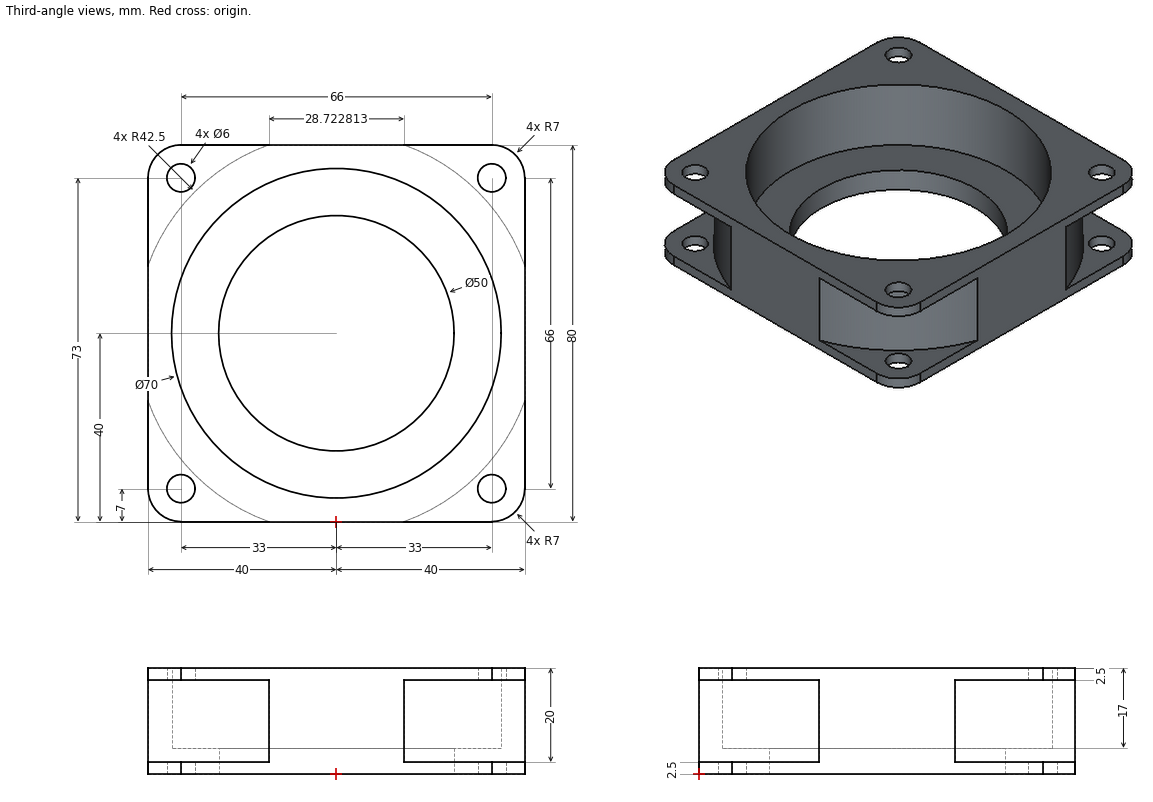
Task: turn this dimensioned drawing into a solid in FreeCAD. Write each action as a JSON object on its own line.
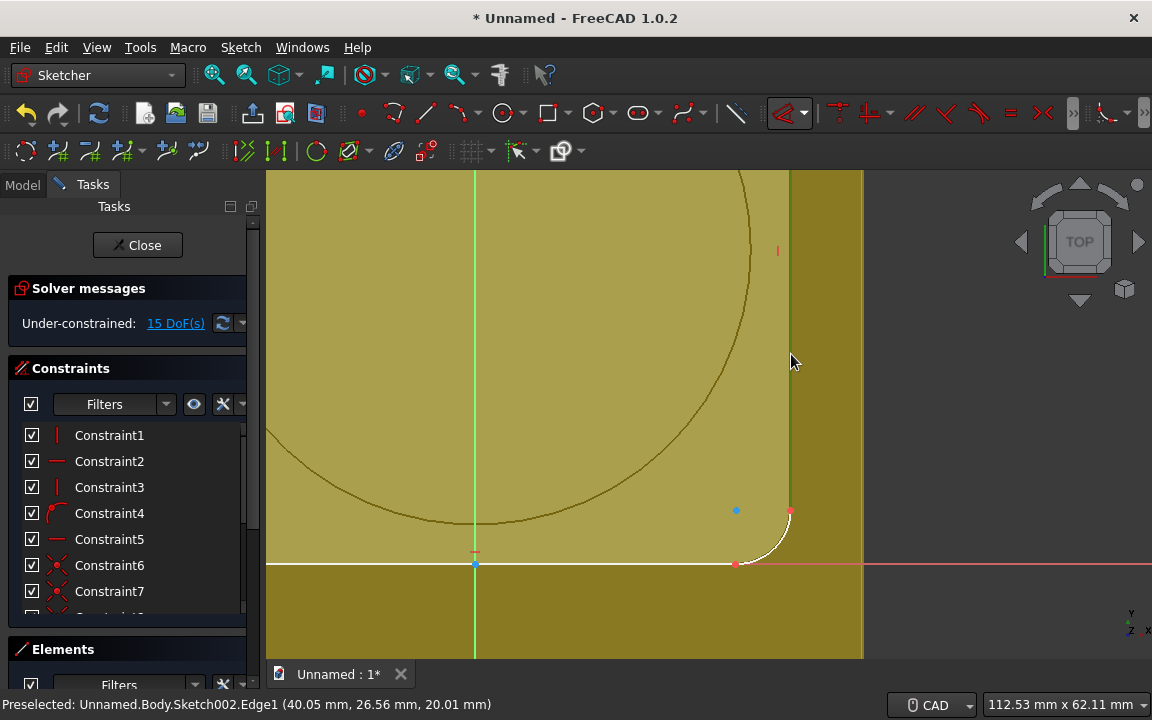
{"action": "scroll", "coordinate": [775, 549], "scroll_direction": "down", "scroll_amount": 4}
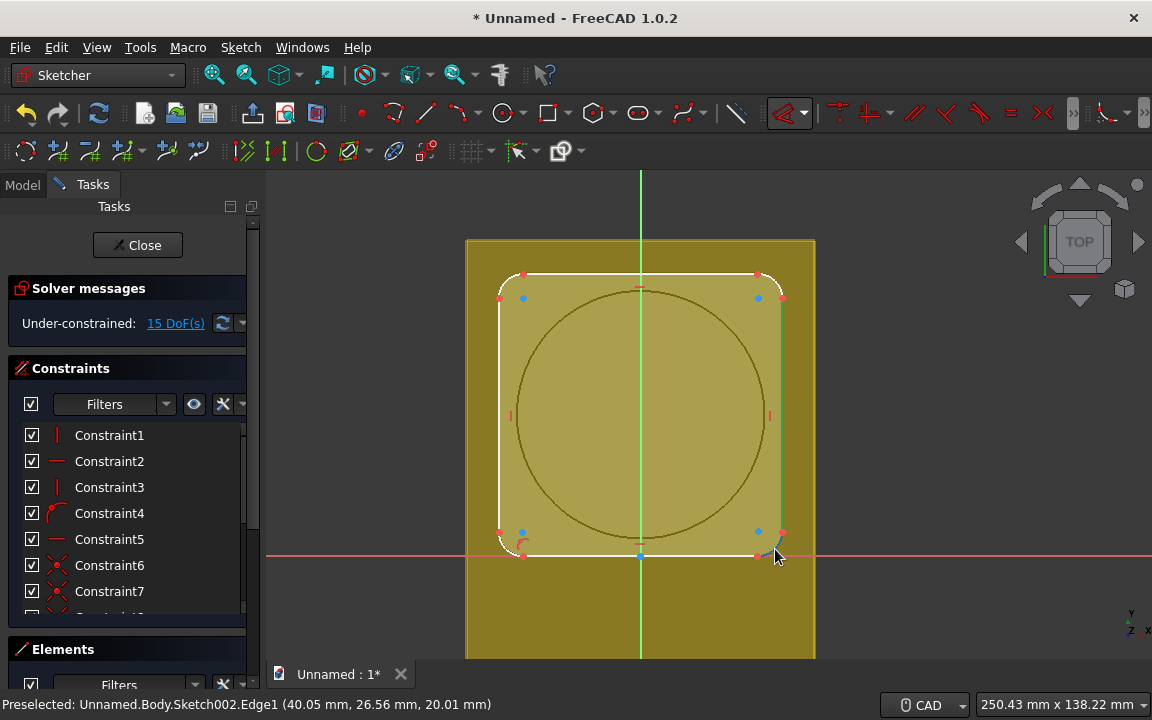
{"action": "left_click", "coordinate": [780, 287]}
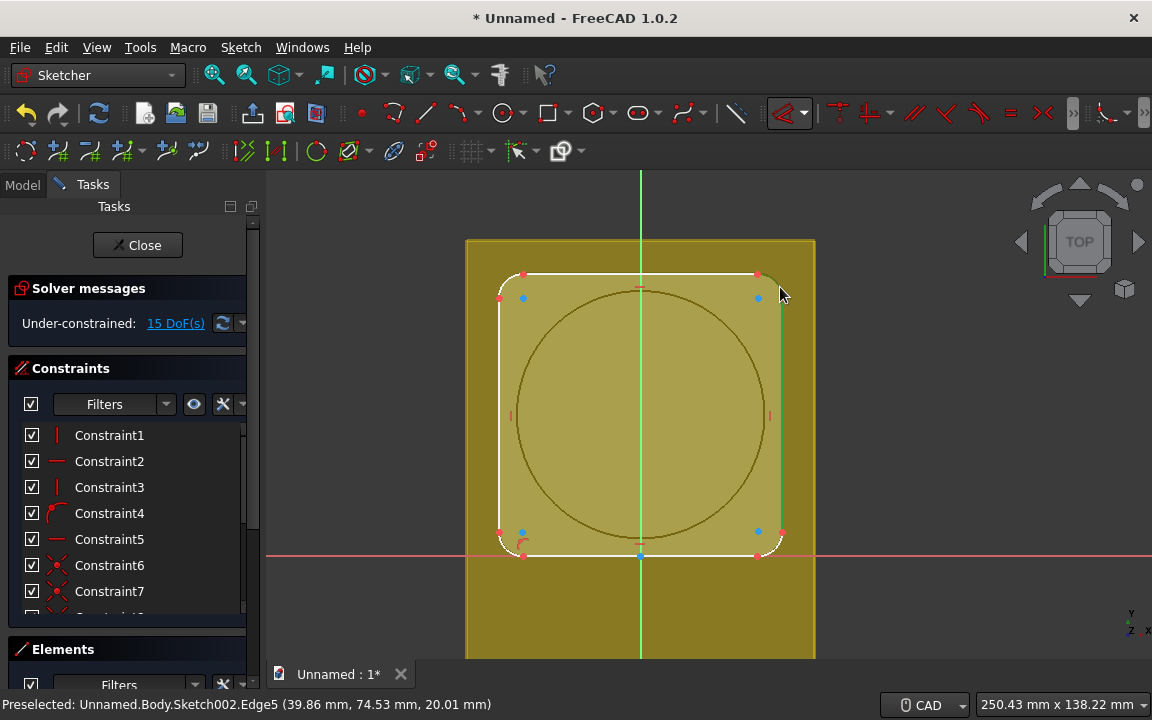
{"action": "left_click", "coordinate": [980, 114]}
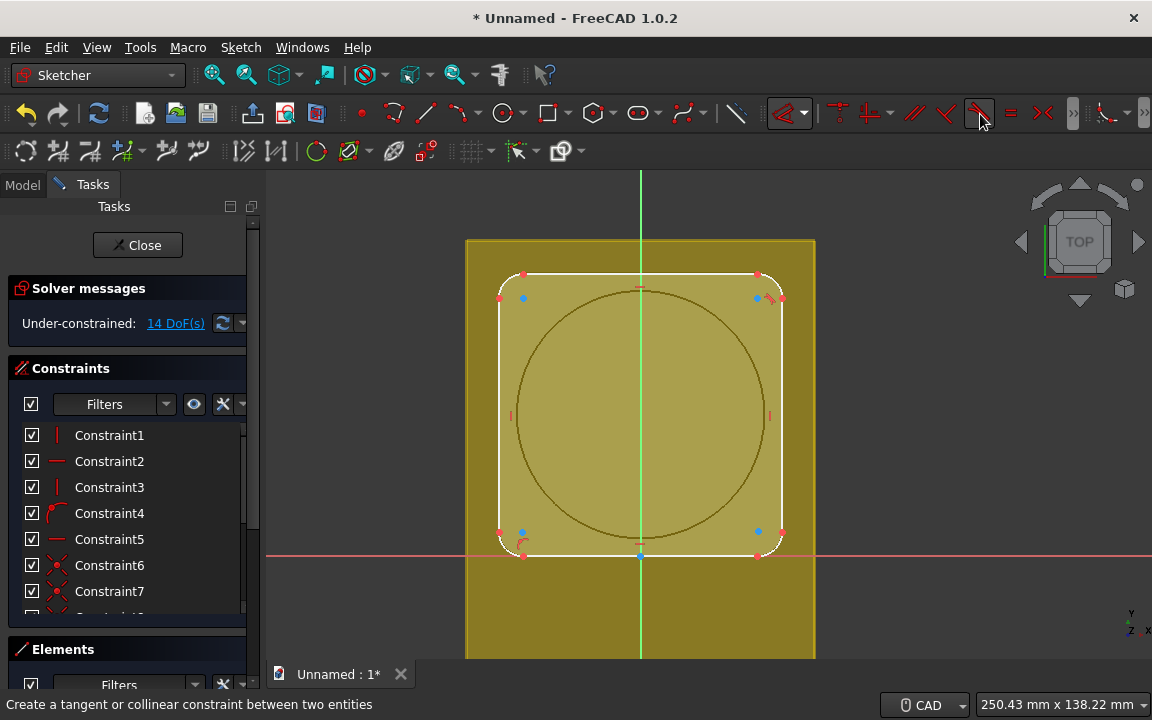
{"action": "left_click", "coordinate": [782, 462]}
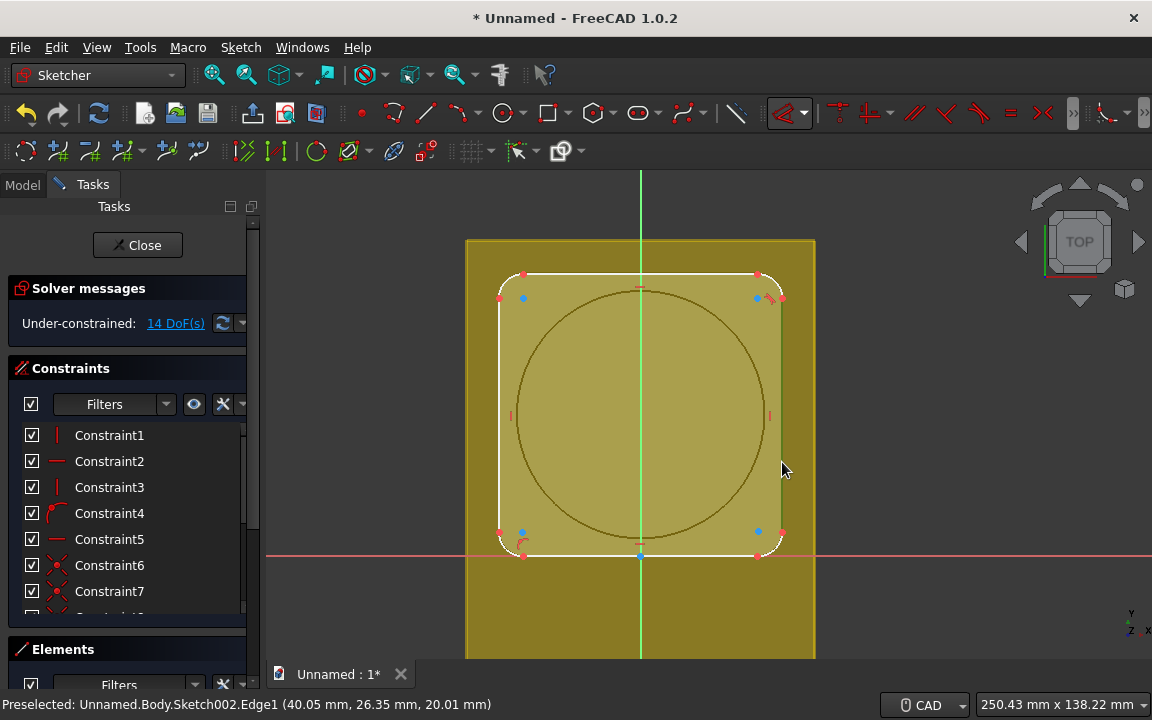
{"action": "left_click", "coordinate": [769, 554]}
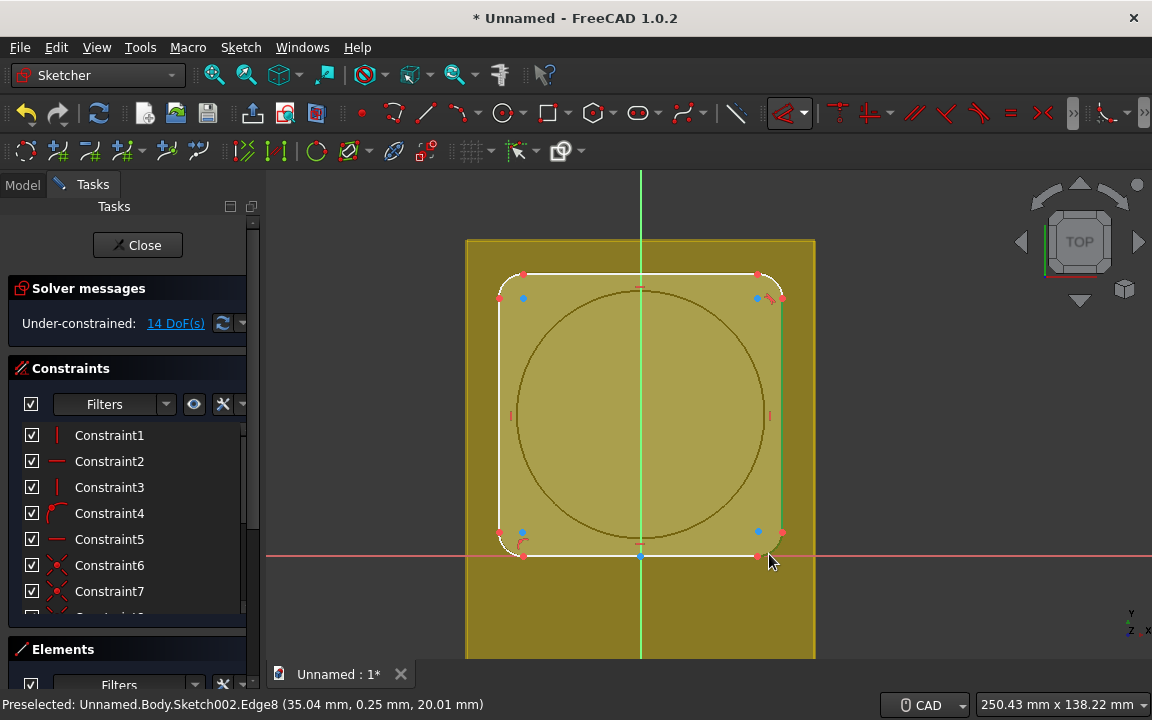
{"action": "left_click", "coordinate": [980, 114]}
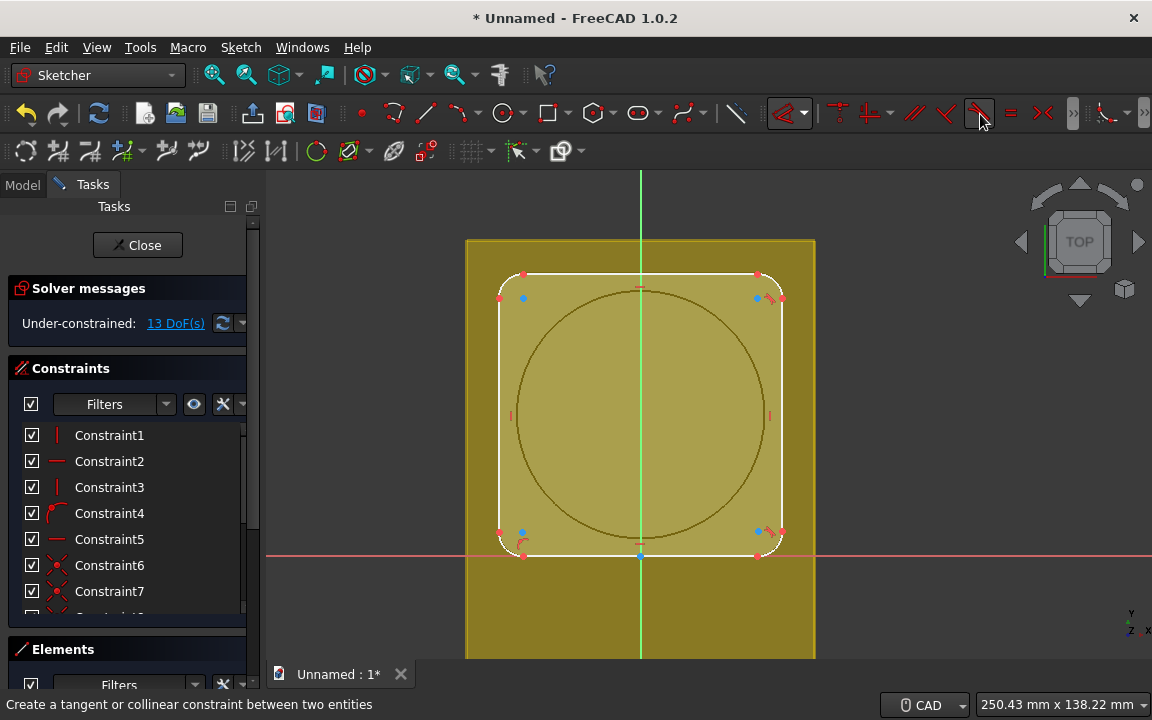
{"action": "left_click", "coordinate": [688, 274]}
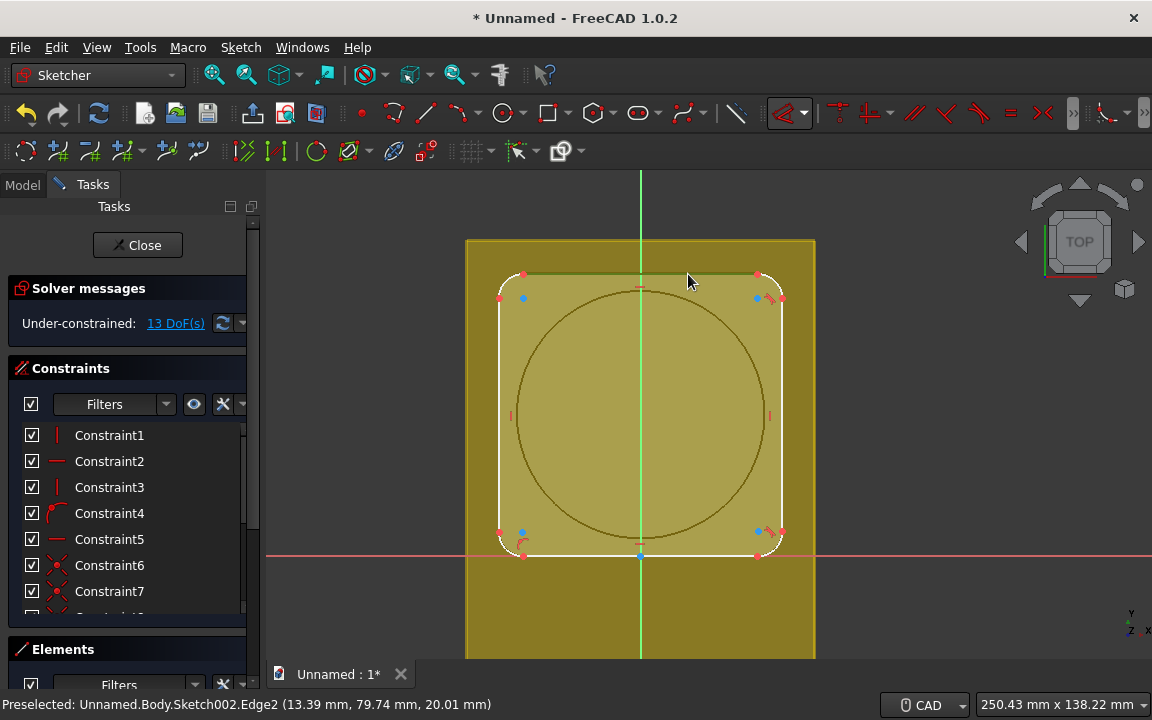
{"action": "left_click", "coordinate": [780, 288]}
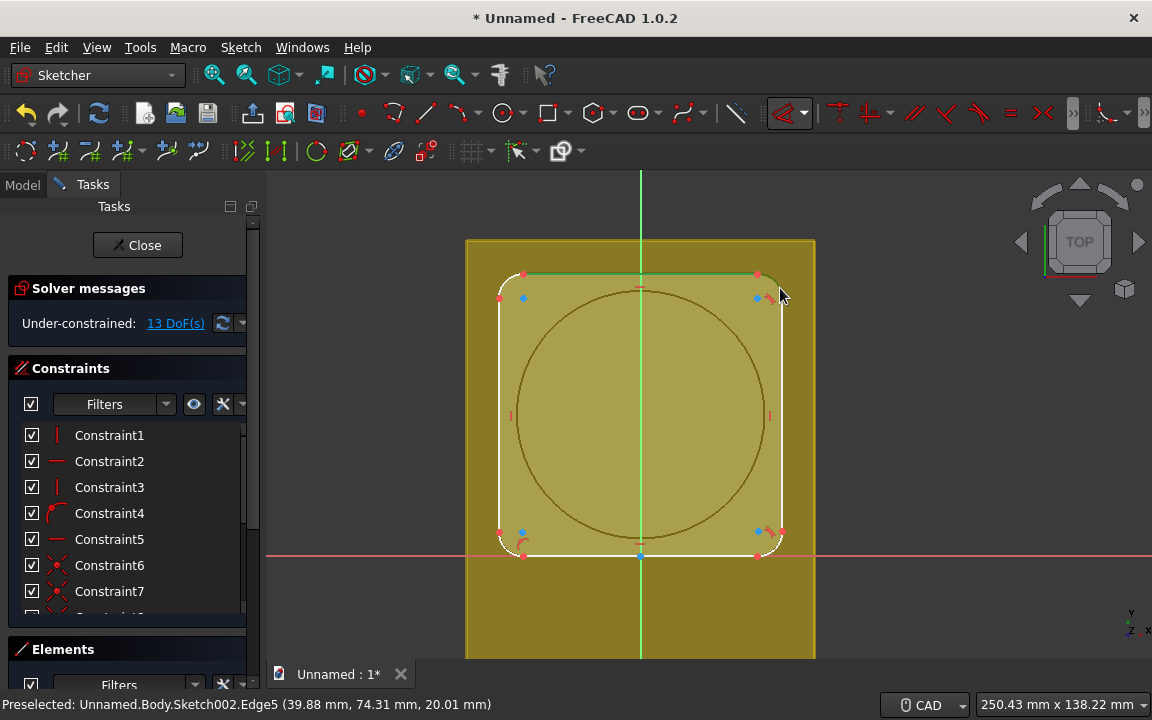
{"action": "key", "text": "t"}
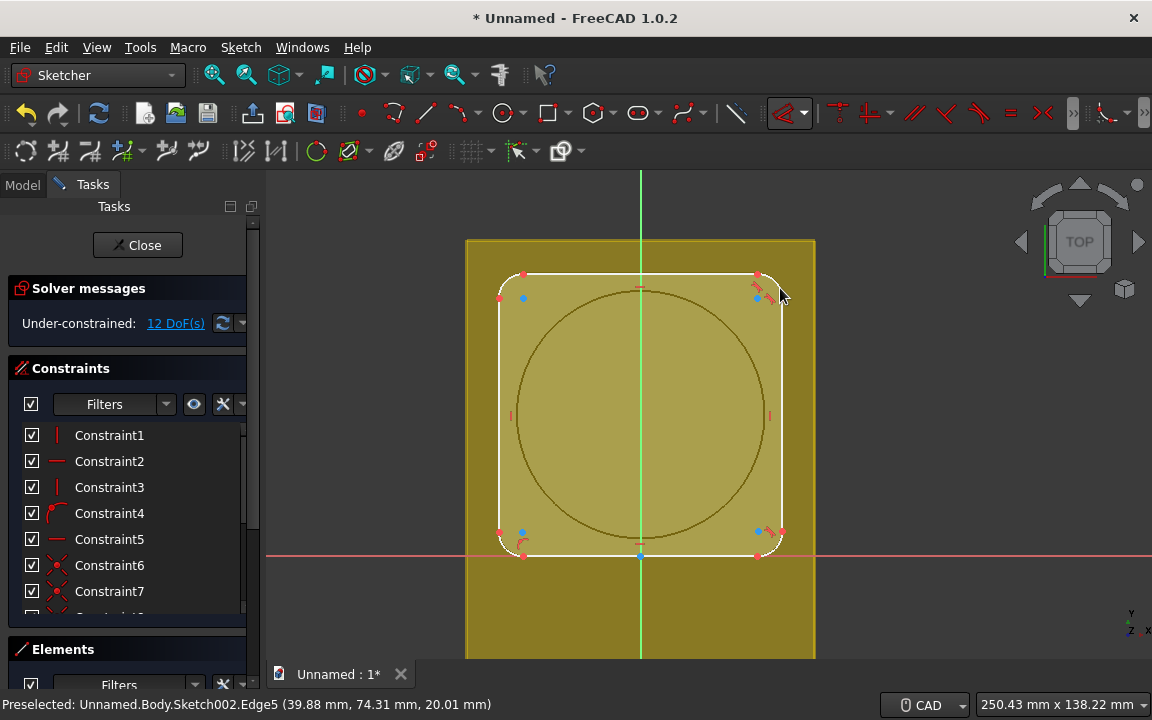
{"action": "left_click", "coordinate": [688, 274]}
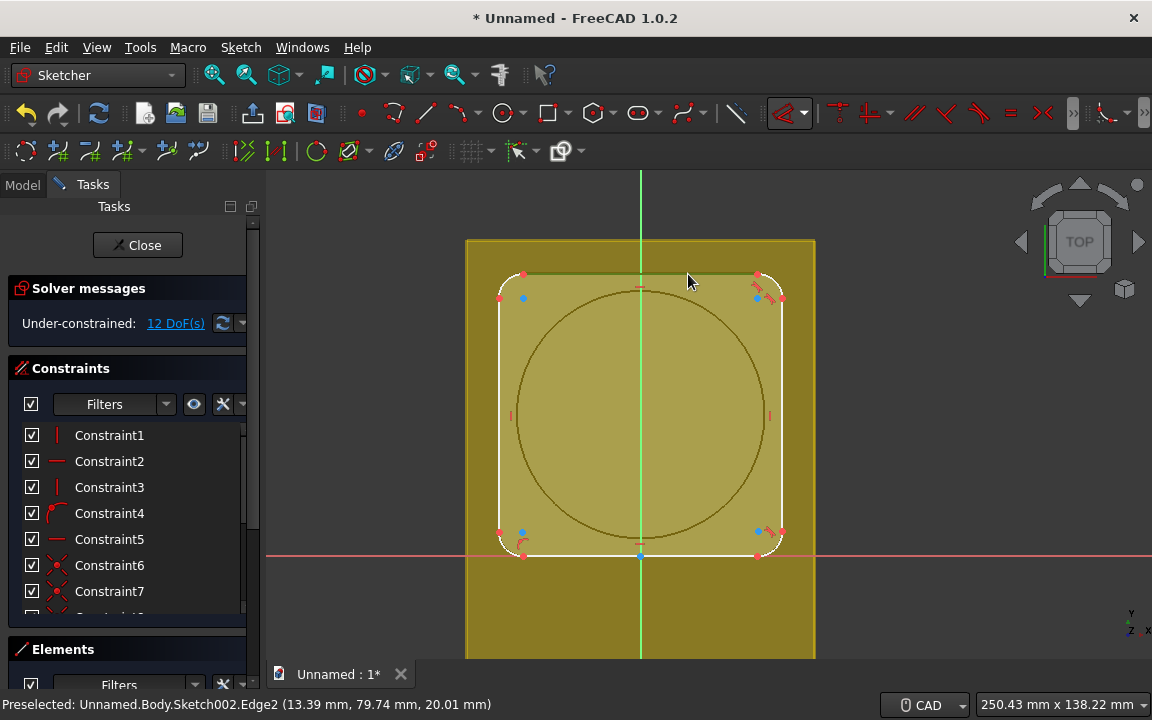
{"action": "left_click", "coordinate": [512, 277]}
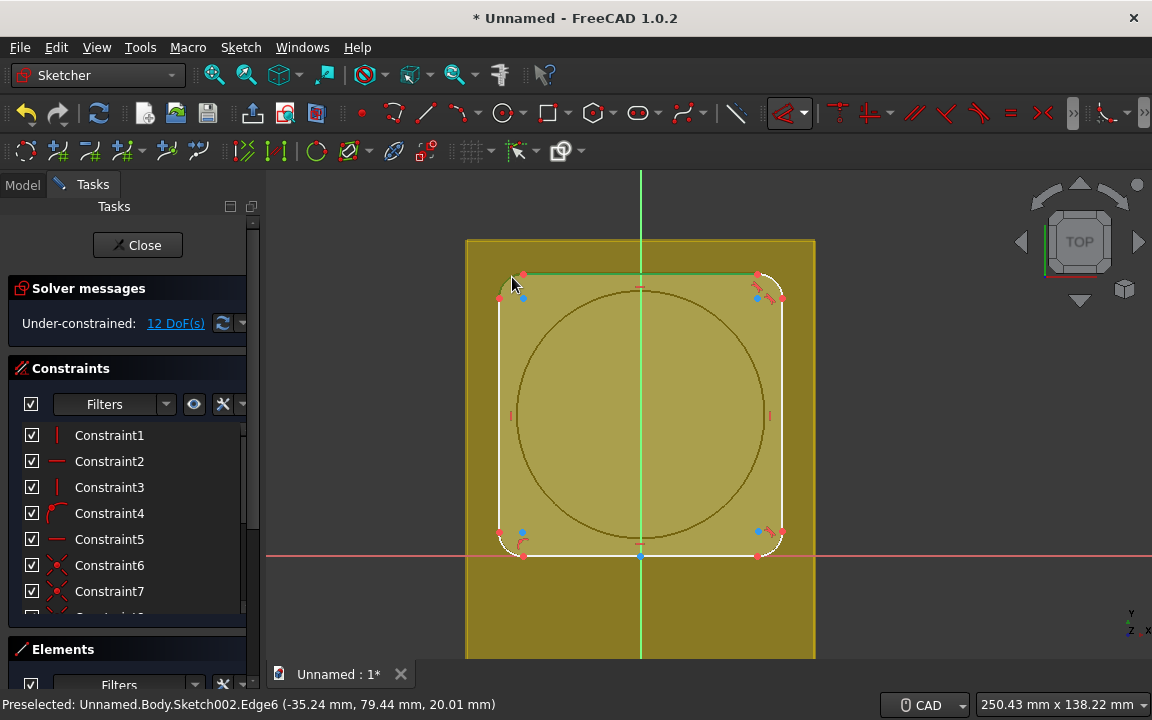
{"action": "key", "text": "t"}